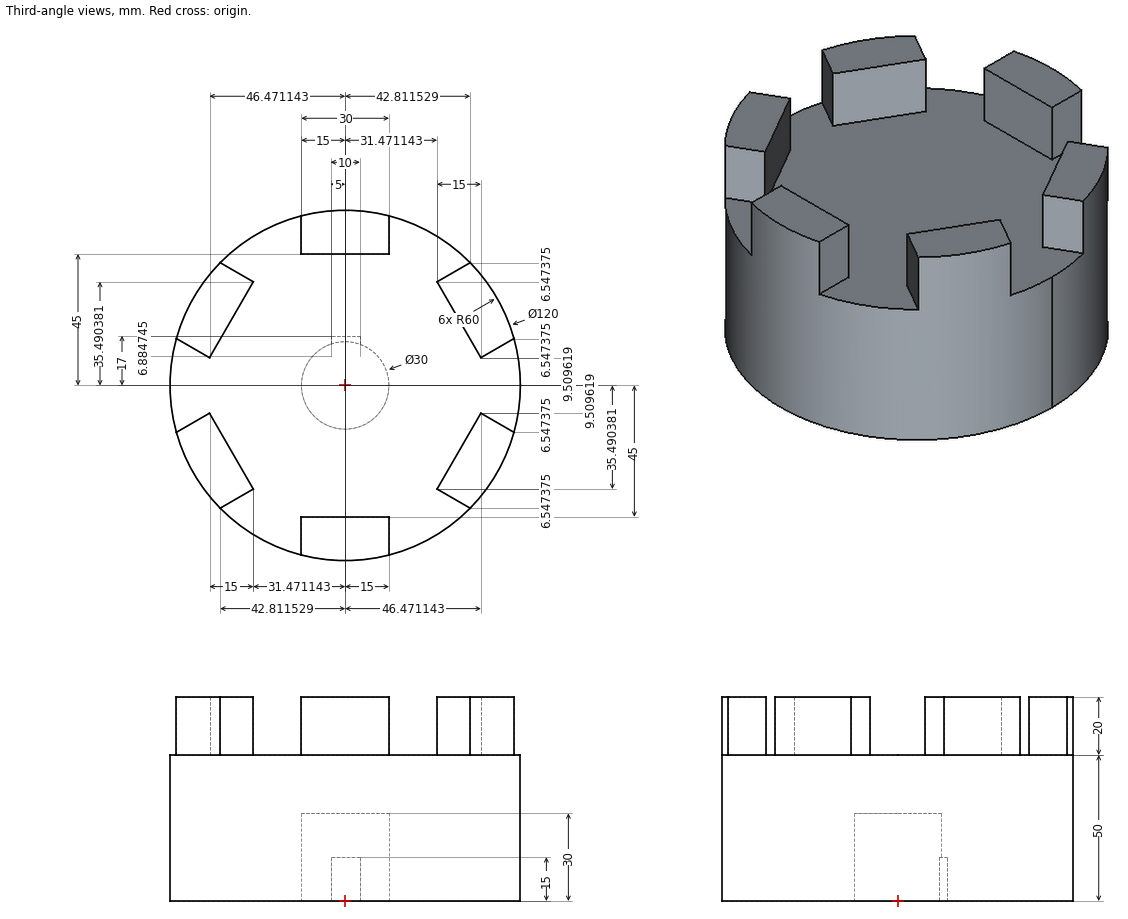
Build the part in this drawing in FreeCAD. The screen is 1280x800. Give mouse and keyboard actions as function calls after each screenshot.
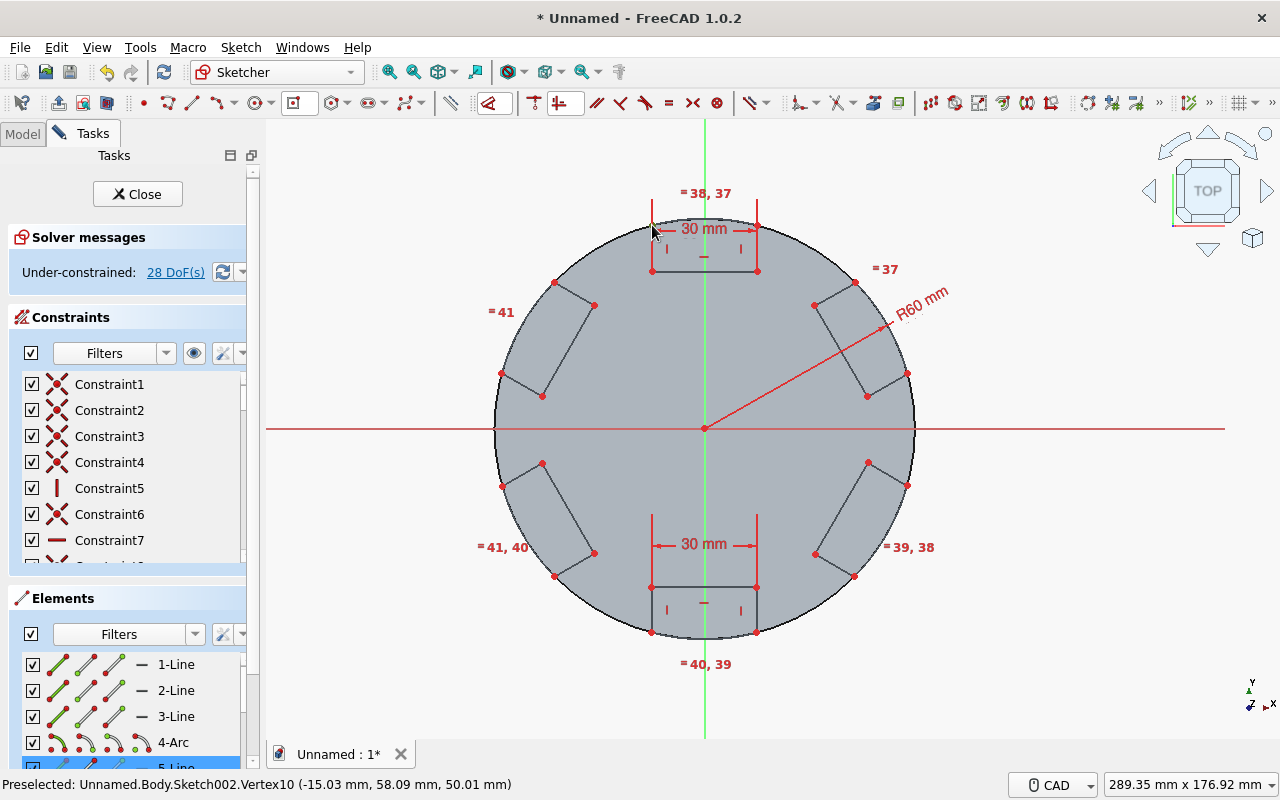
key(l)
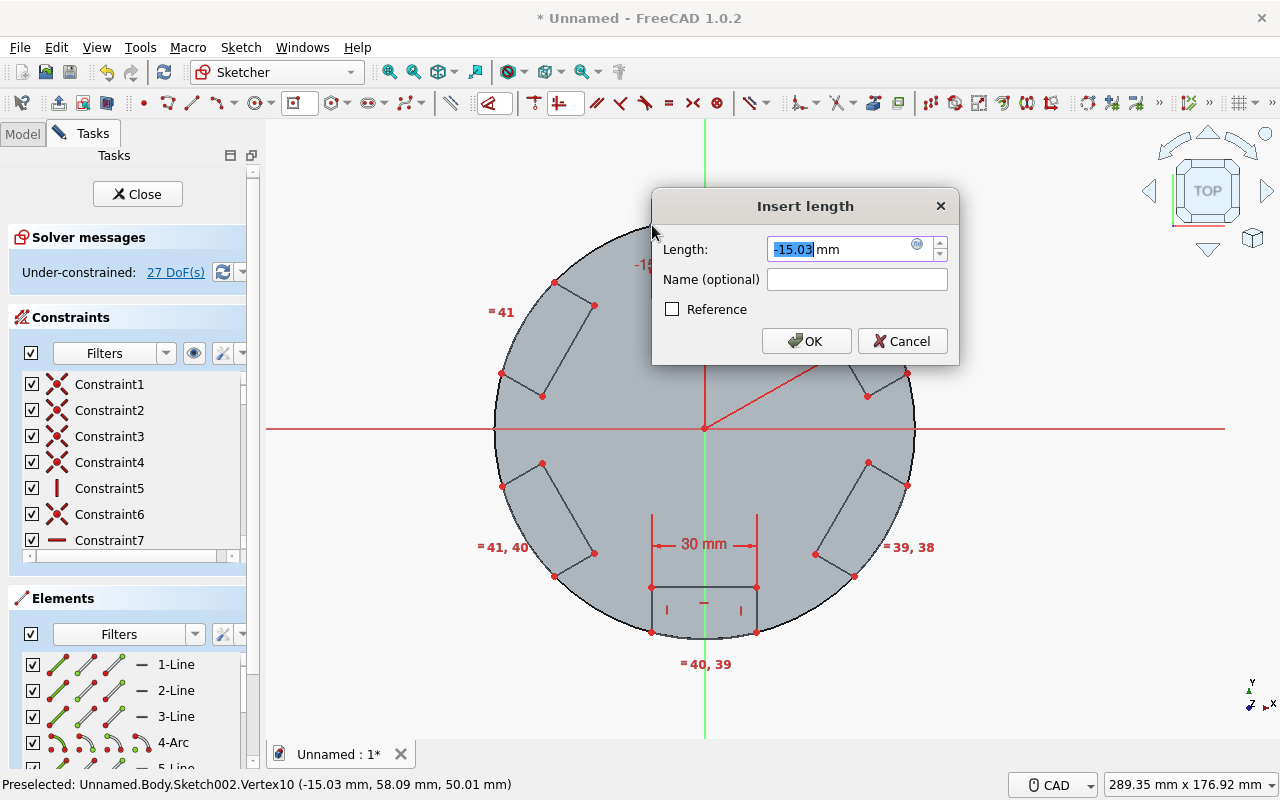
text(-15)
key(Return)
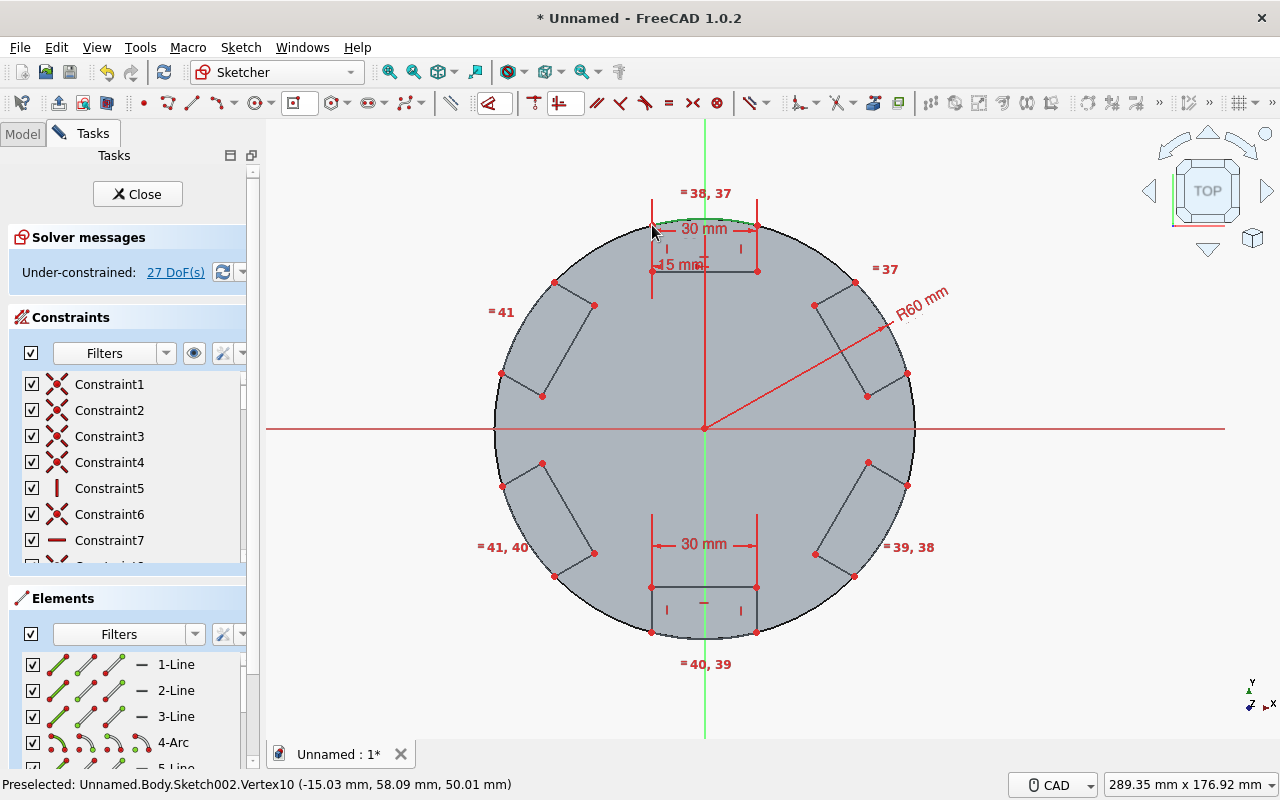
click(652, 272)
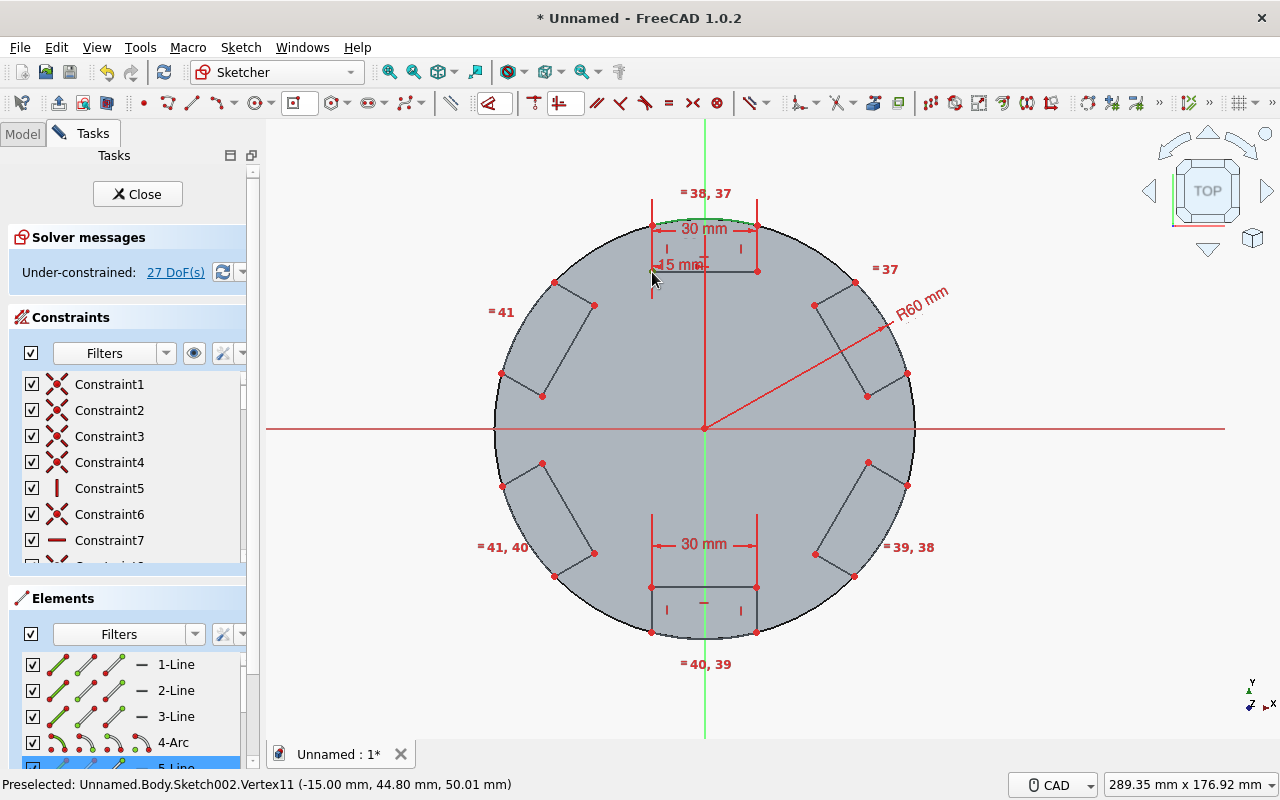
click(506, 104)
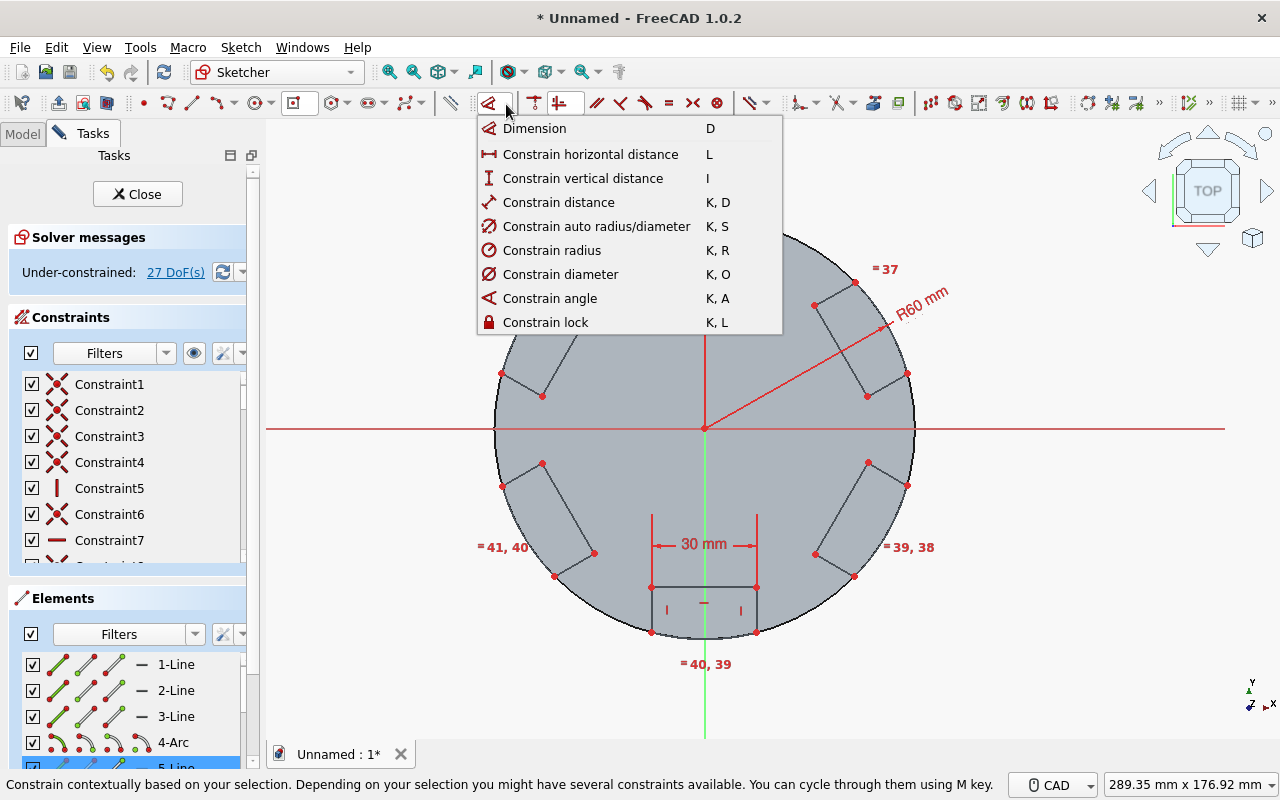
click(630, 178)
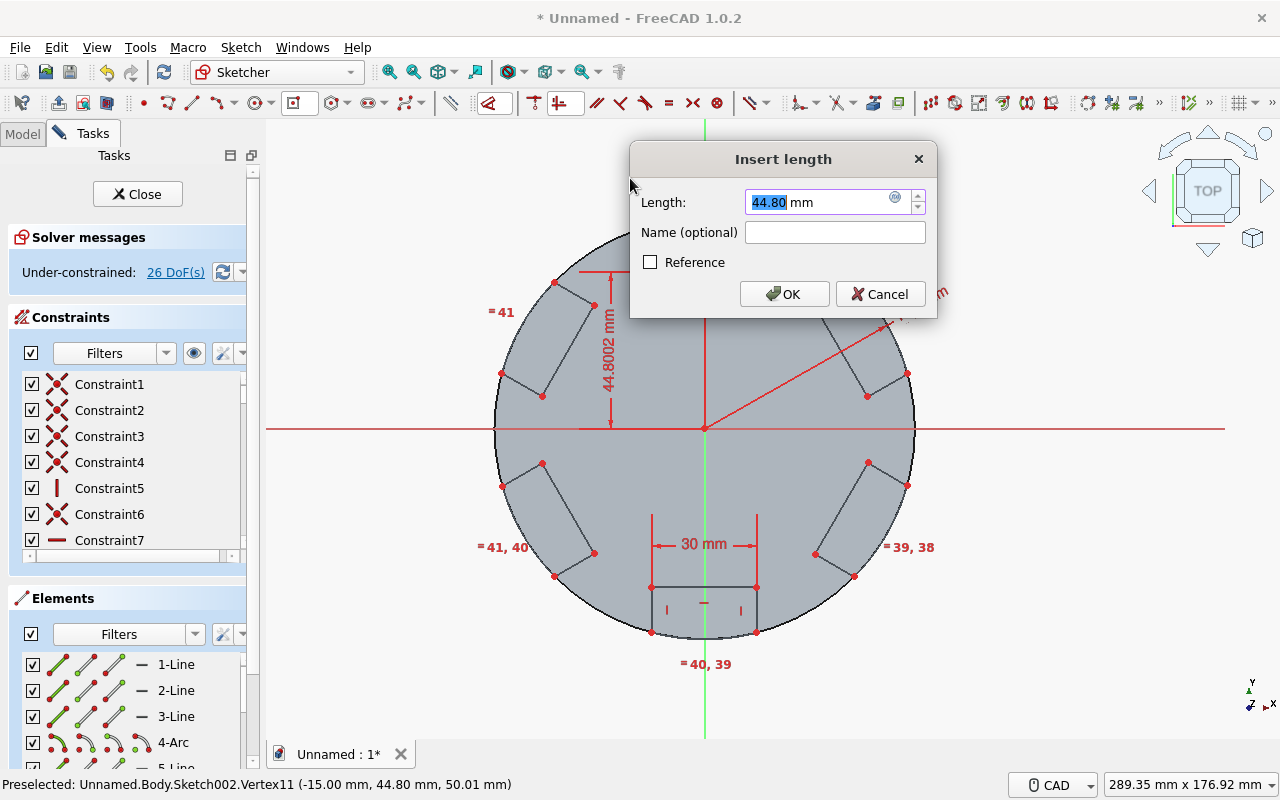
text(45)
key(Return)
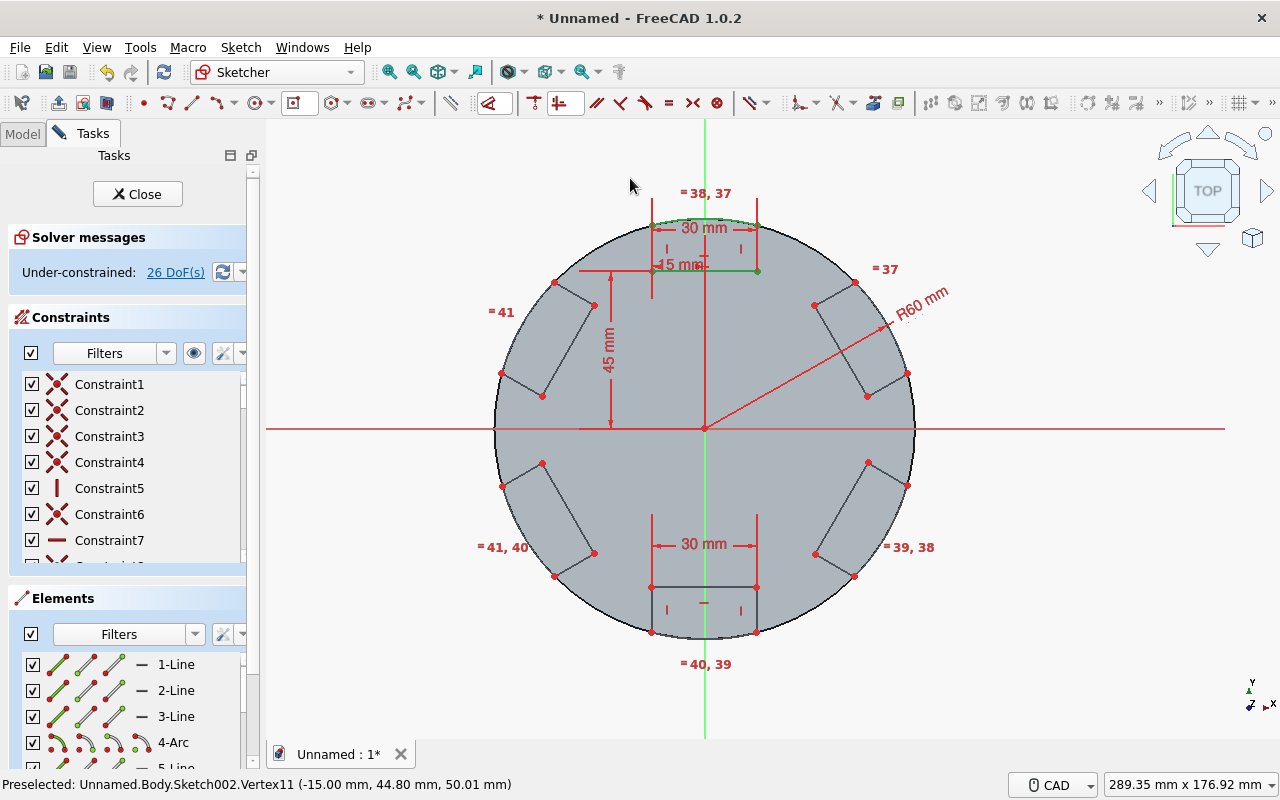
click(757, 633)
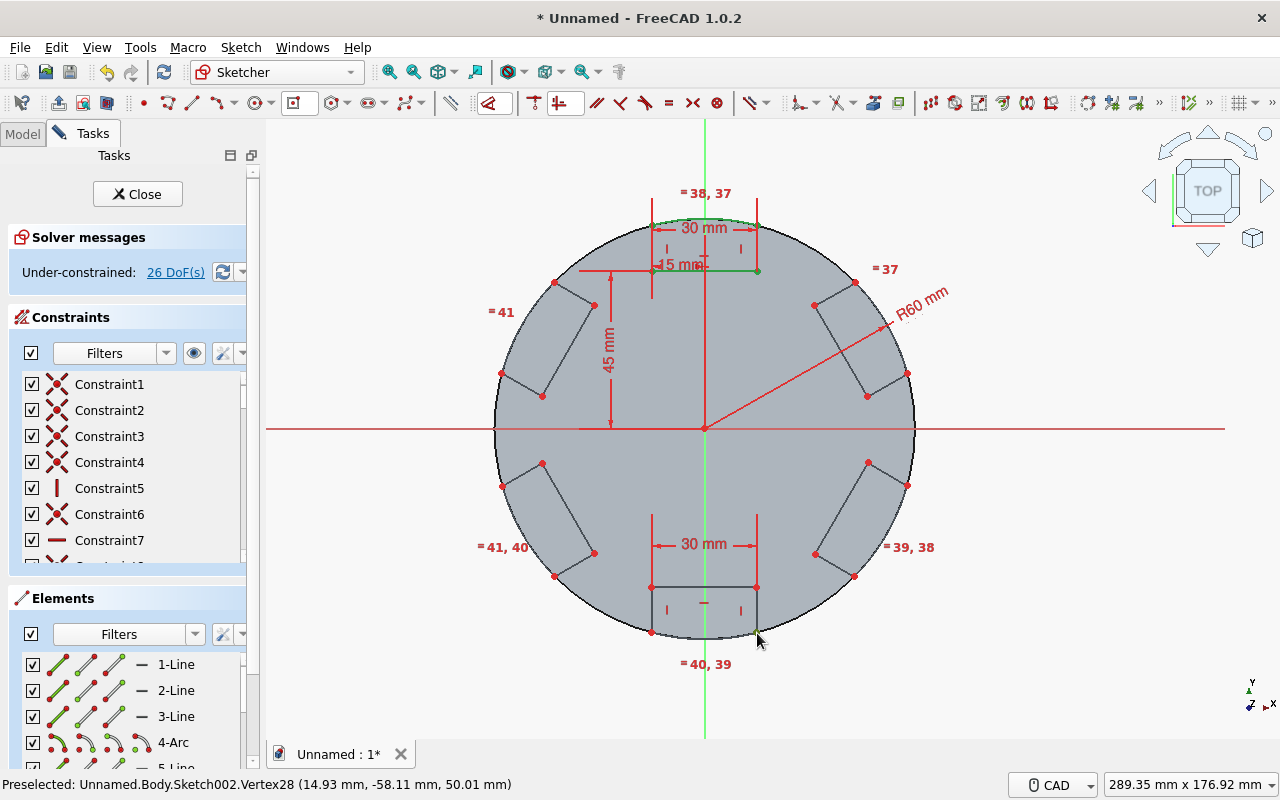
click(506, 104)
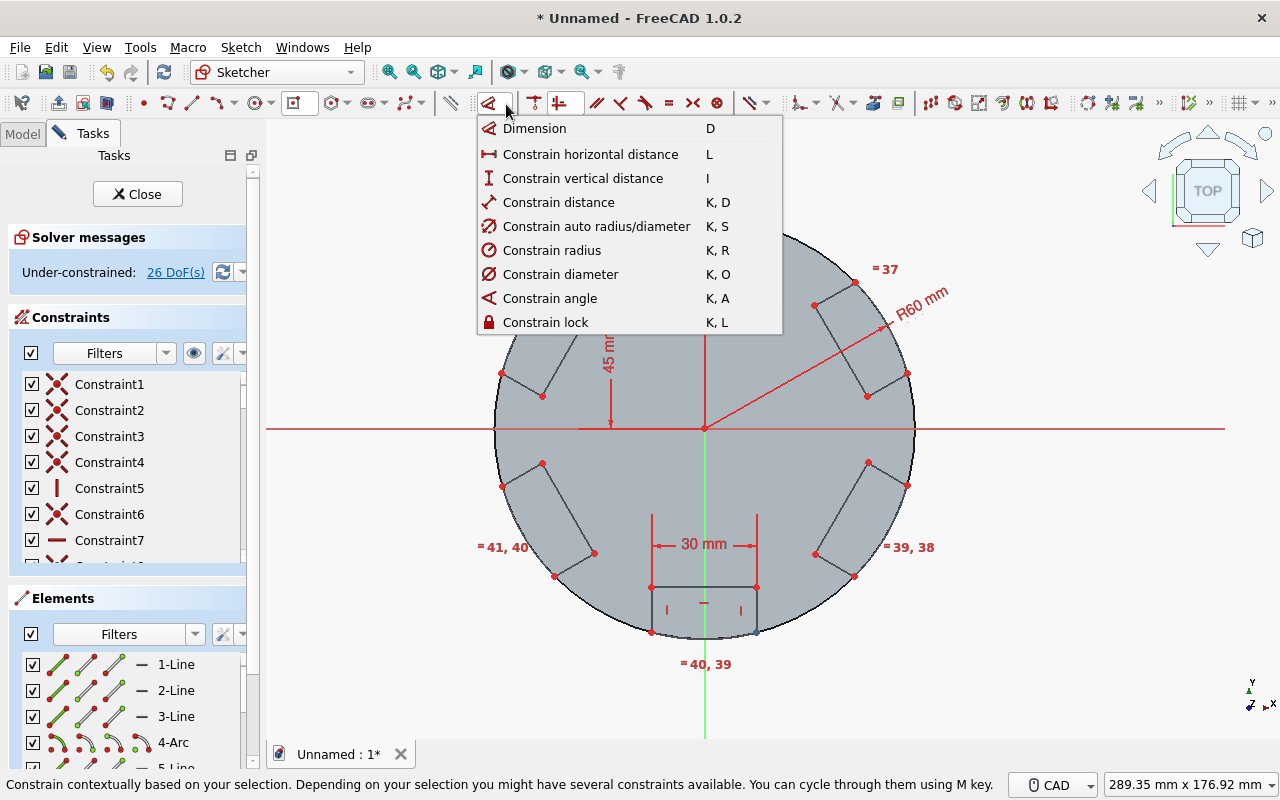
click(630, 154)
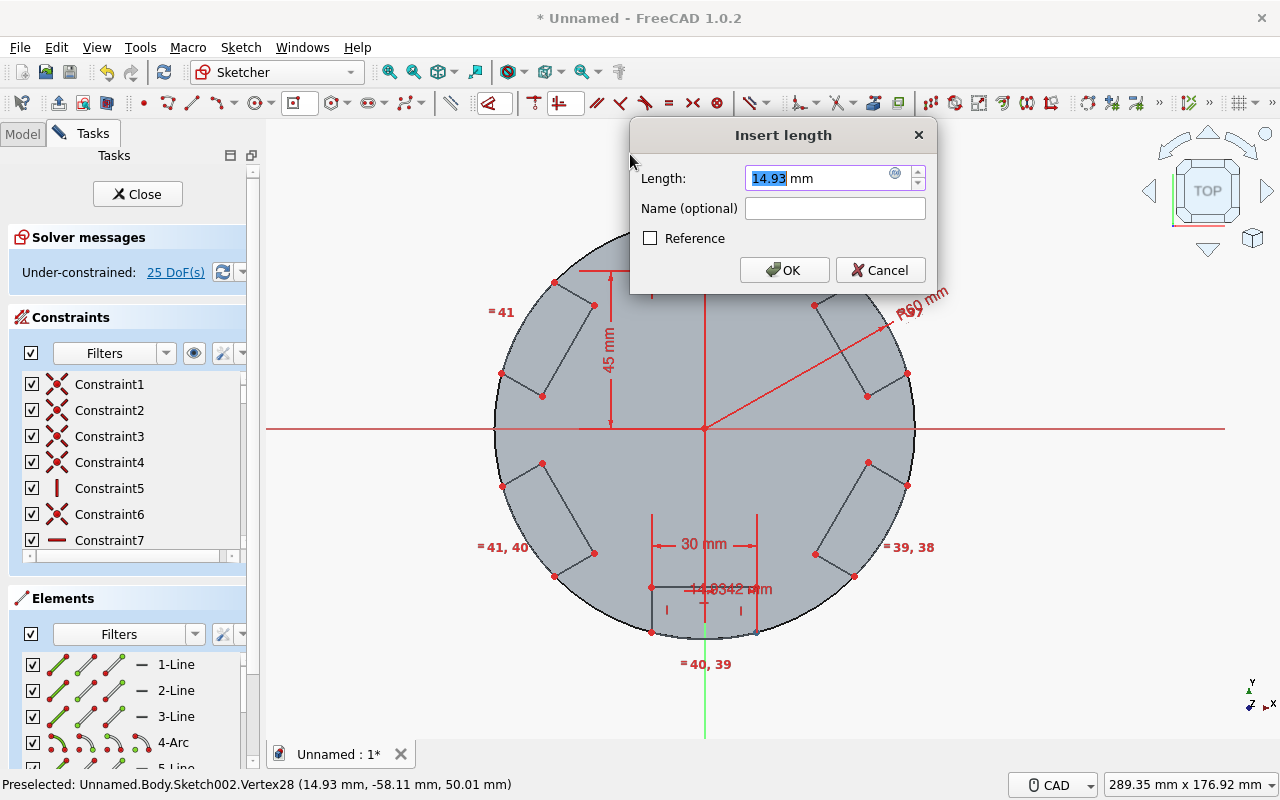
text(15)
key(Return)